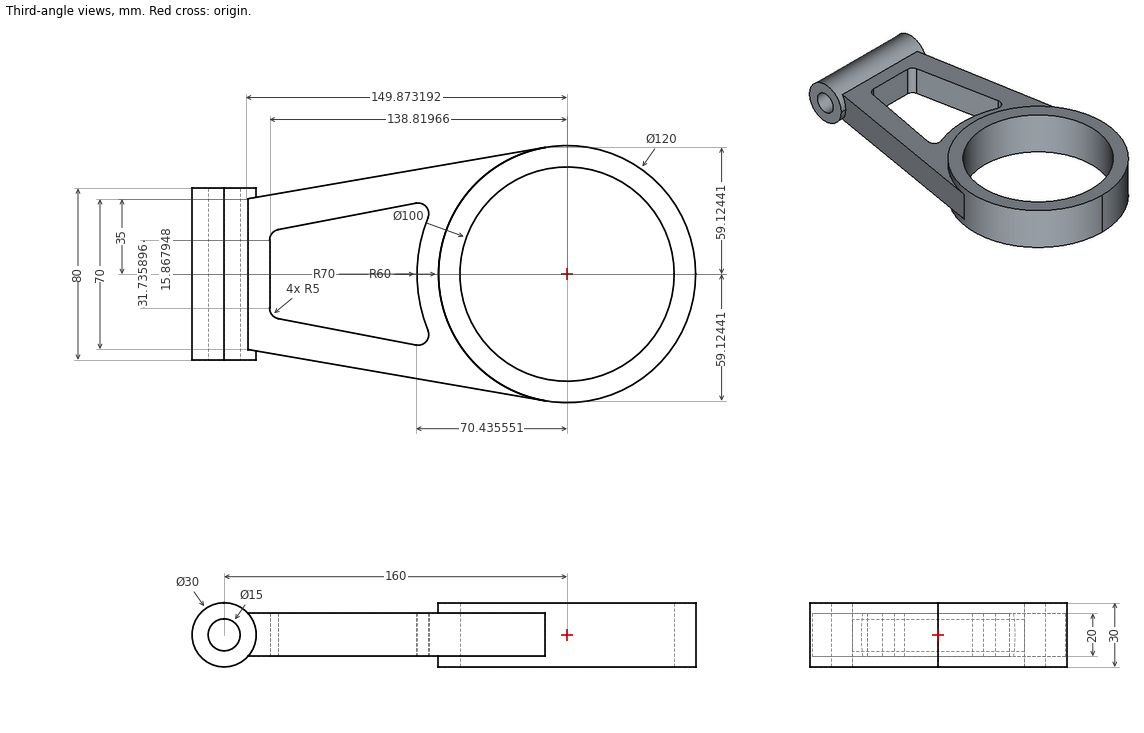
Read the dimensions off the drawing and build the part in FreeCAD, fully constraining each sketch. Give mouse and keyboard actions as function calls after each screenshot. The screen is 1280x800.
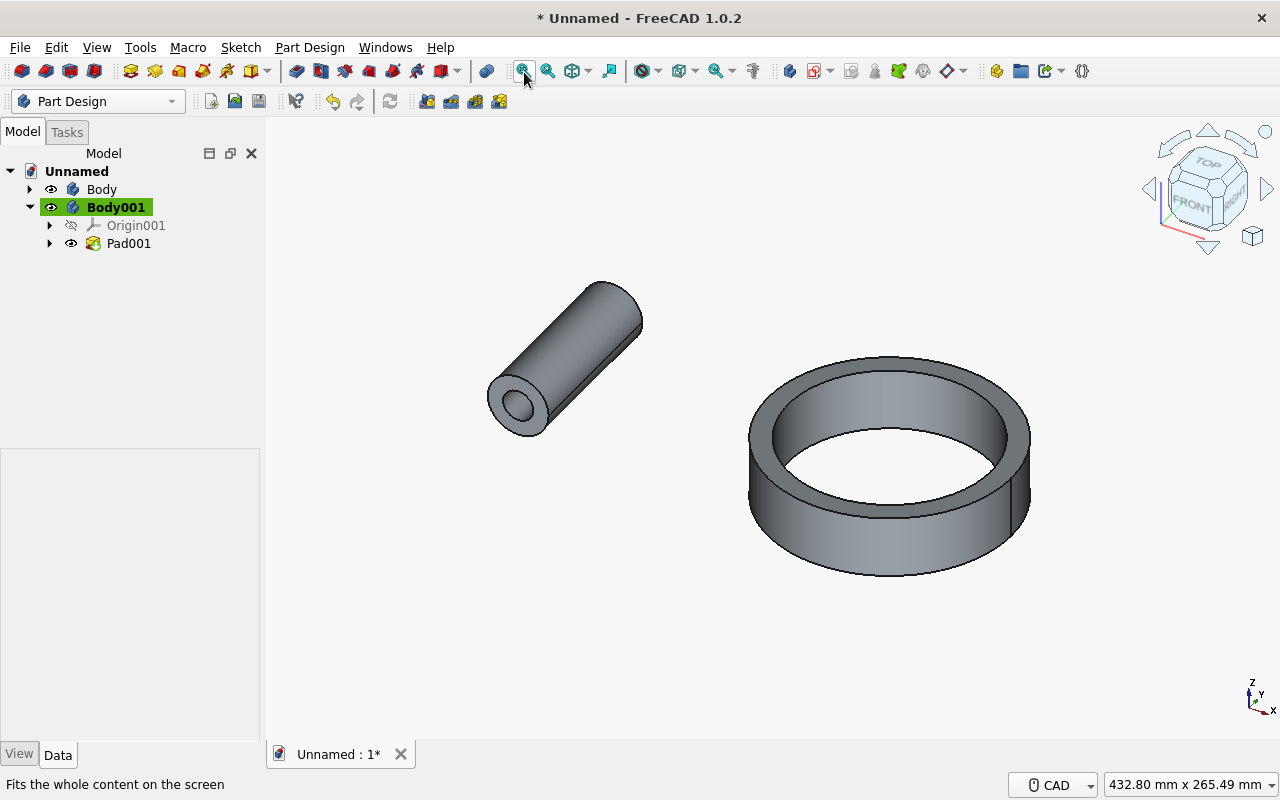
double_click(96, 189)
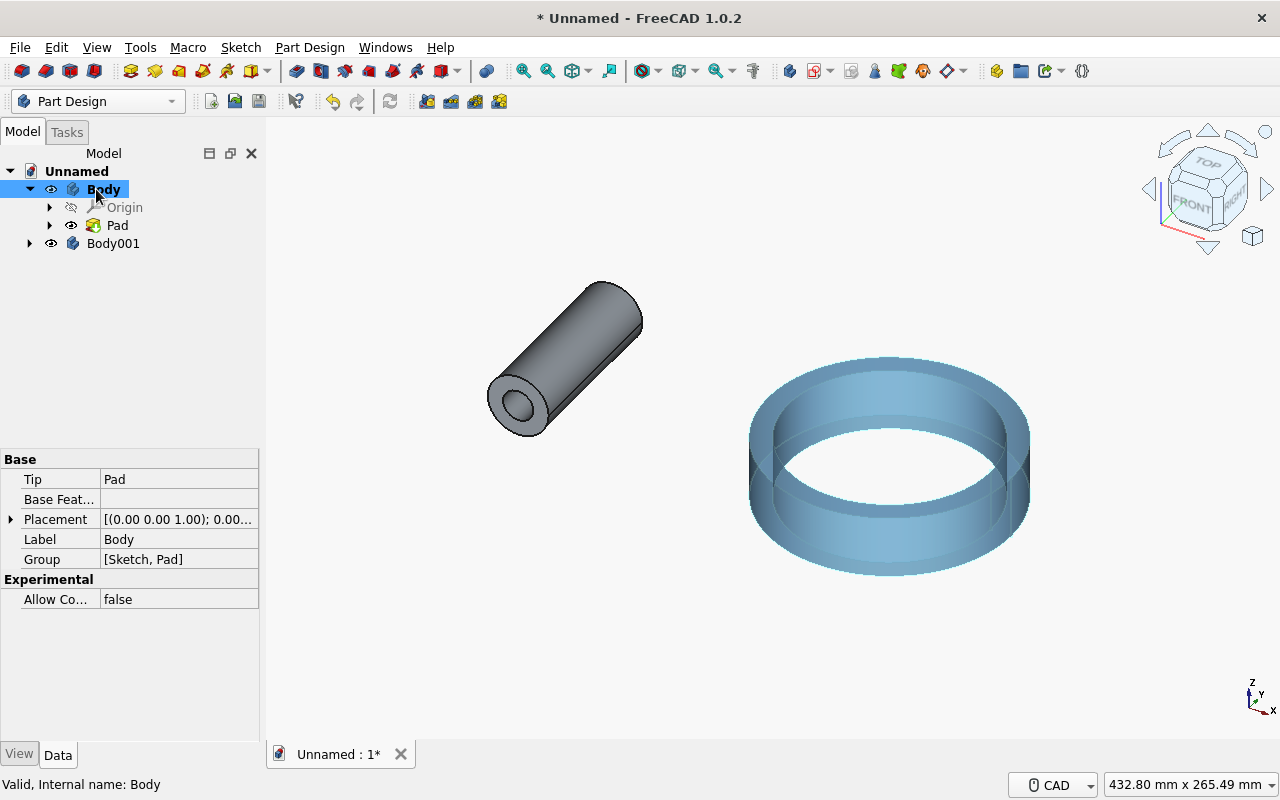
click(96, 189)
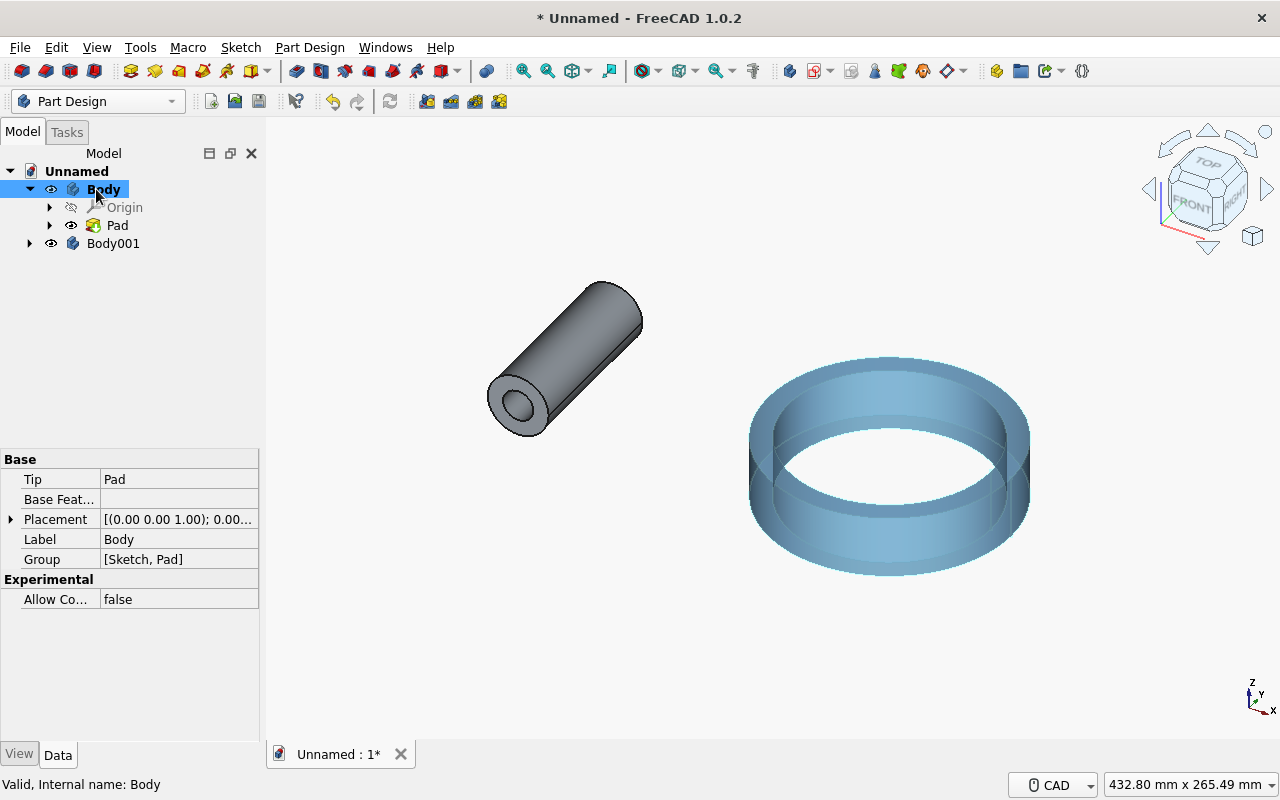
click(146, 599)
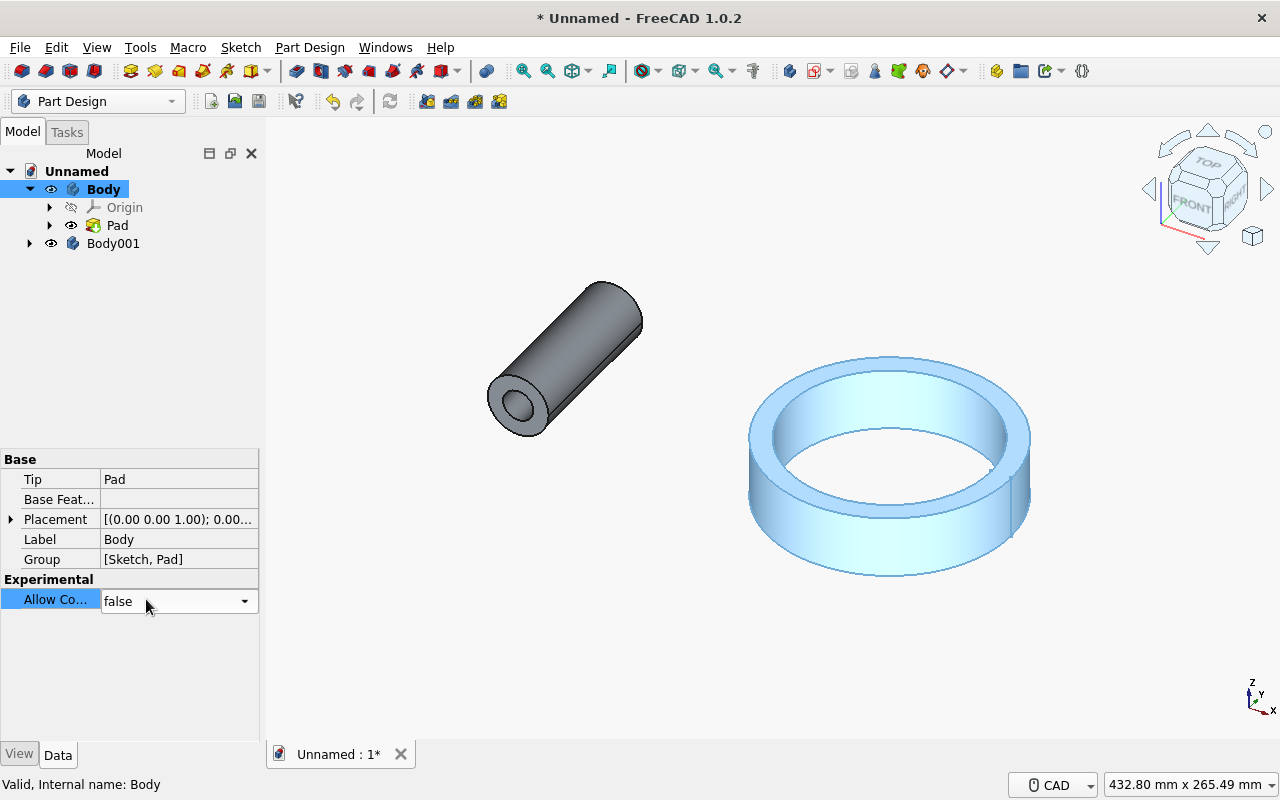
click(146, 599)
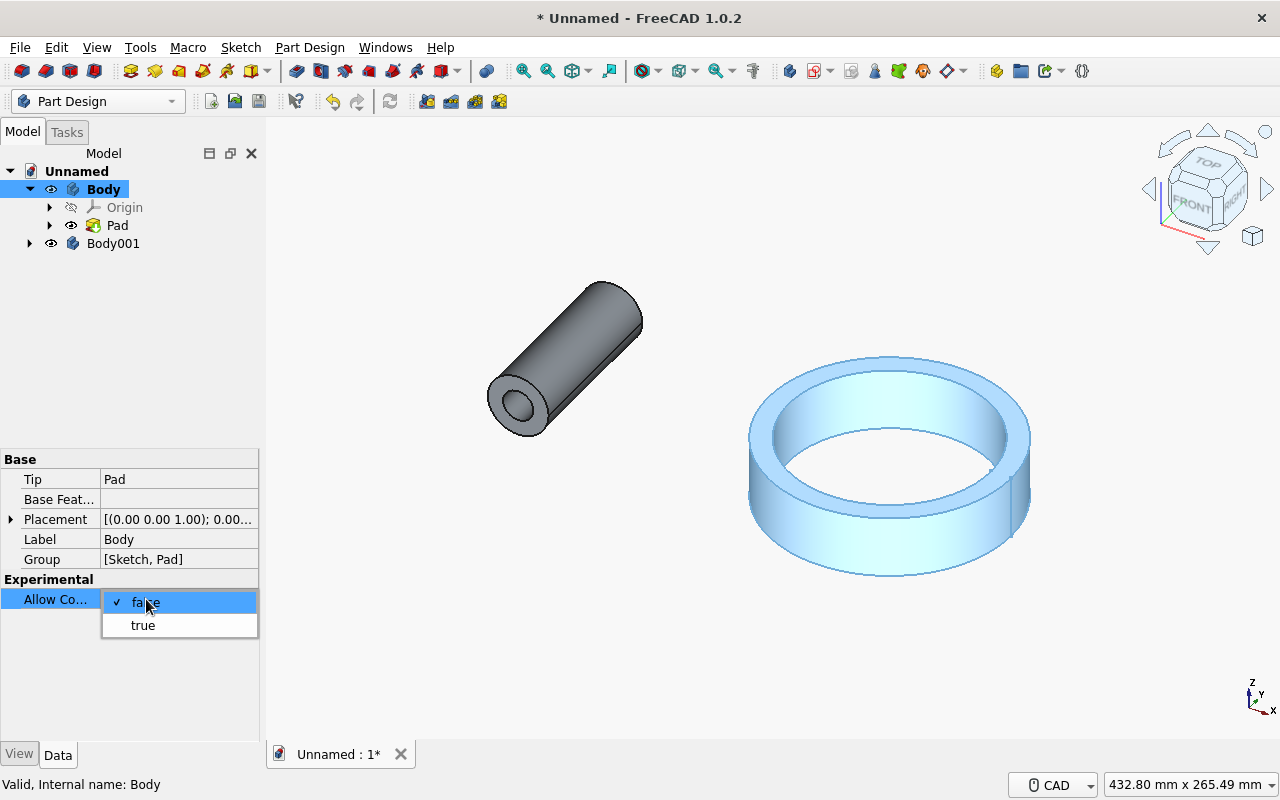
click(179, 626)
key(Return)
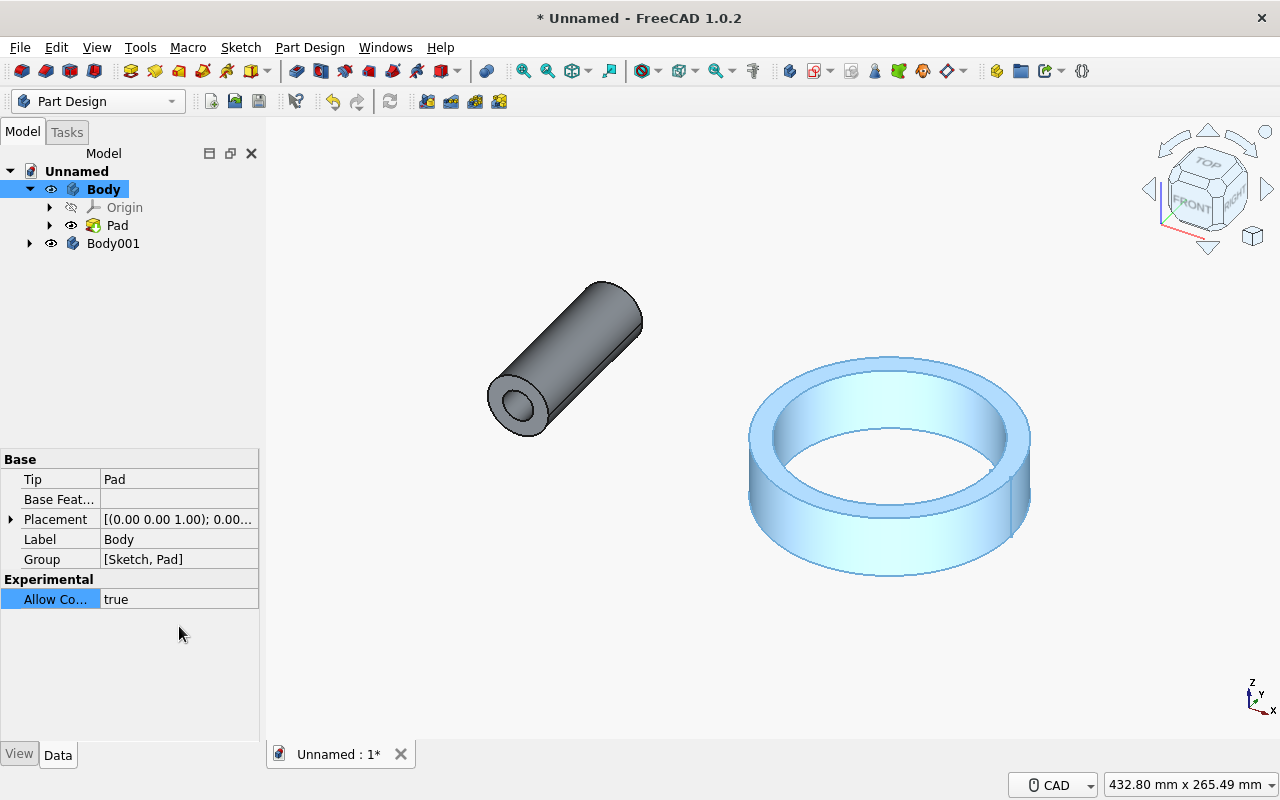
click(96, 243)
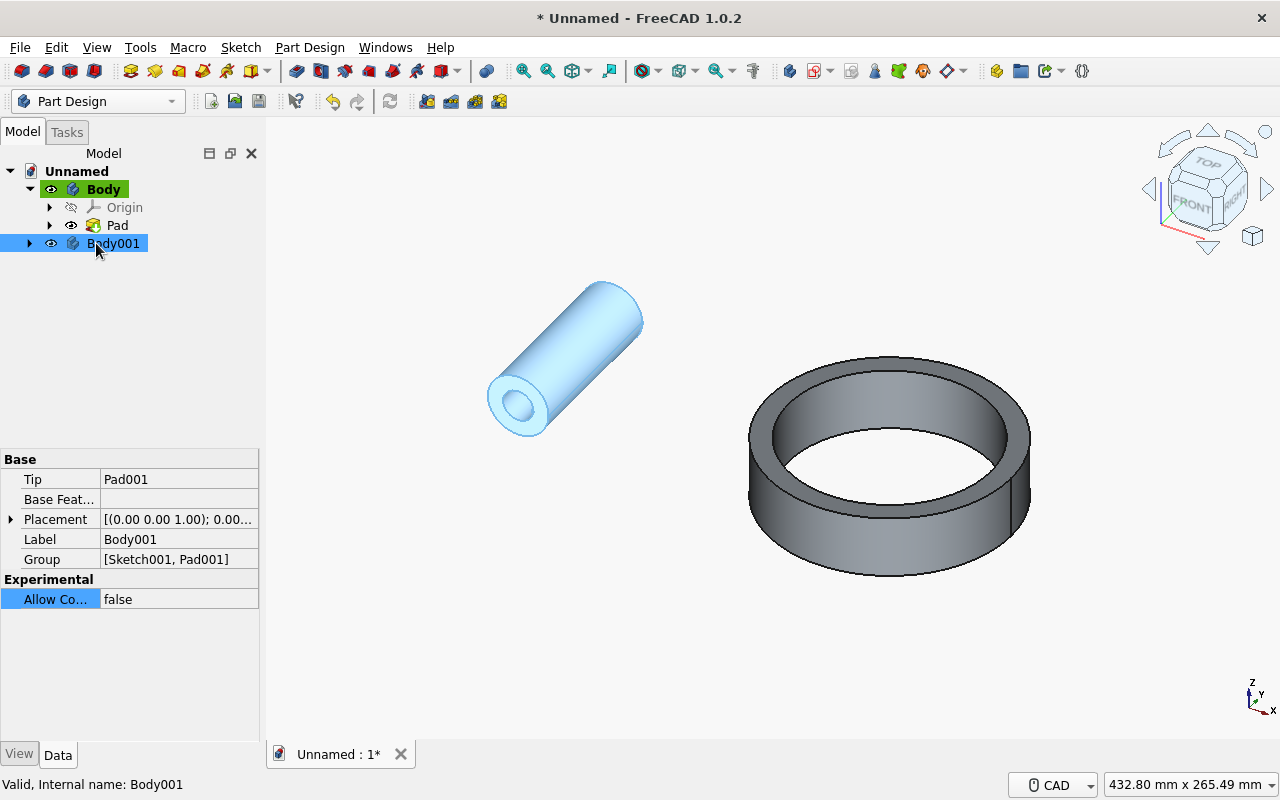
click(488, 72)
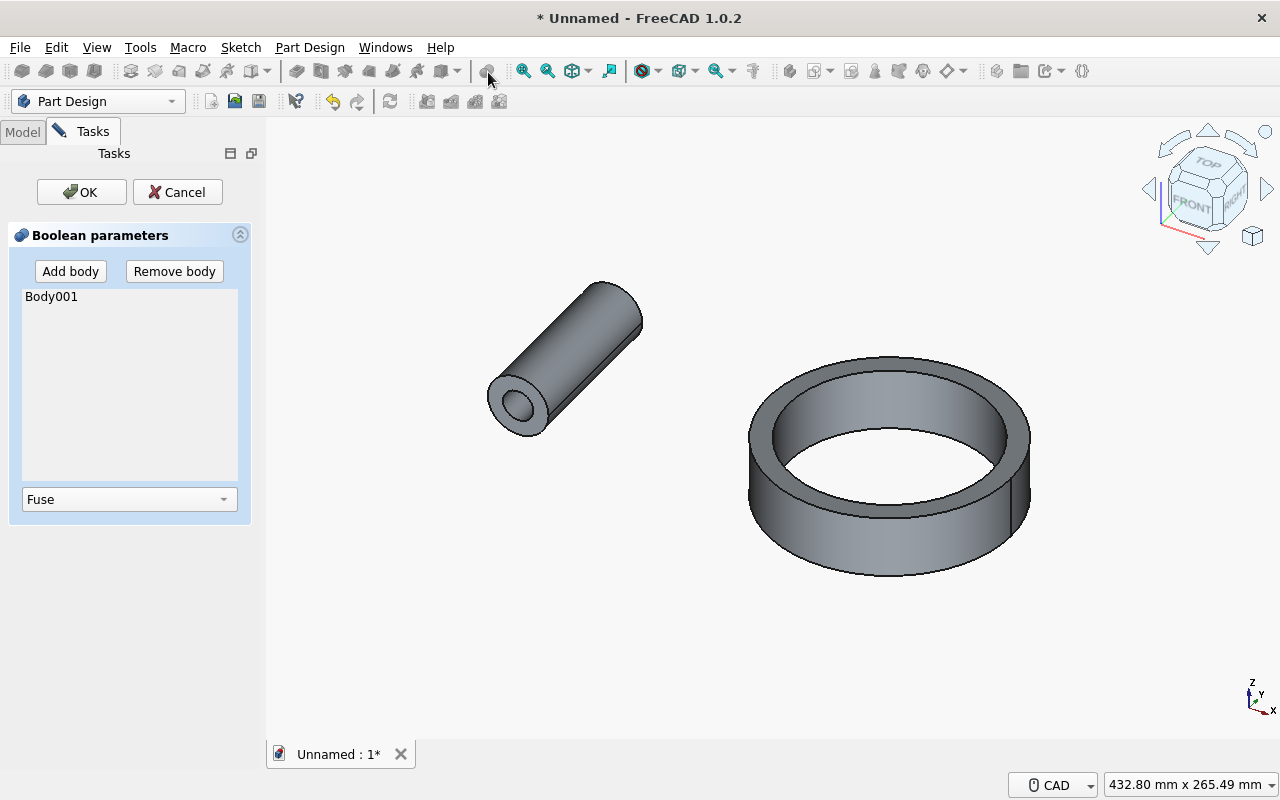
click(82, 192)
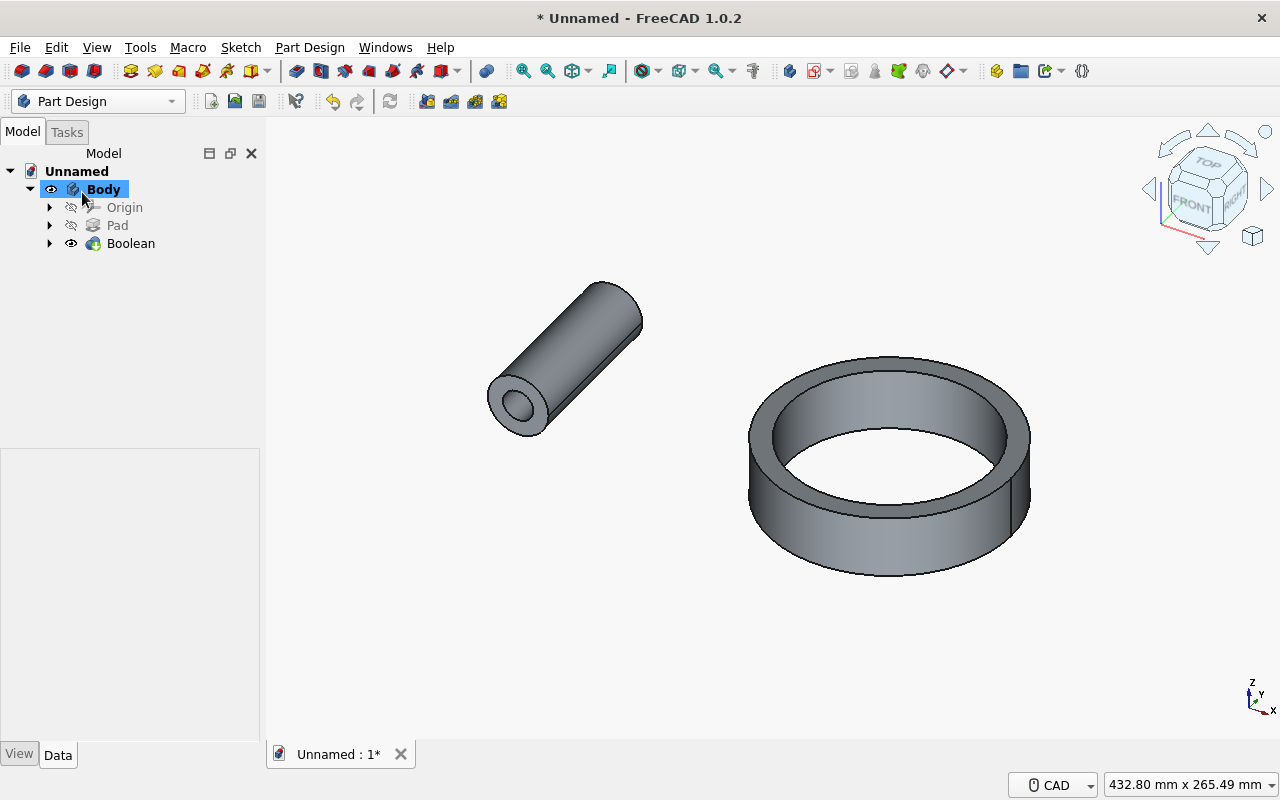
click(814, 72)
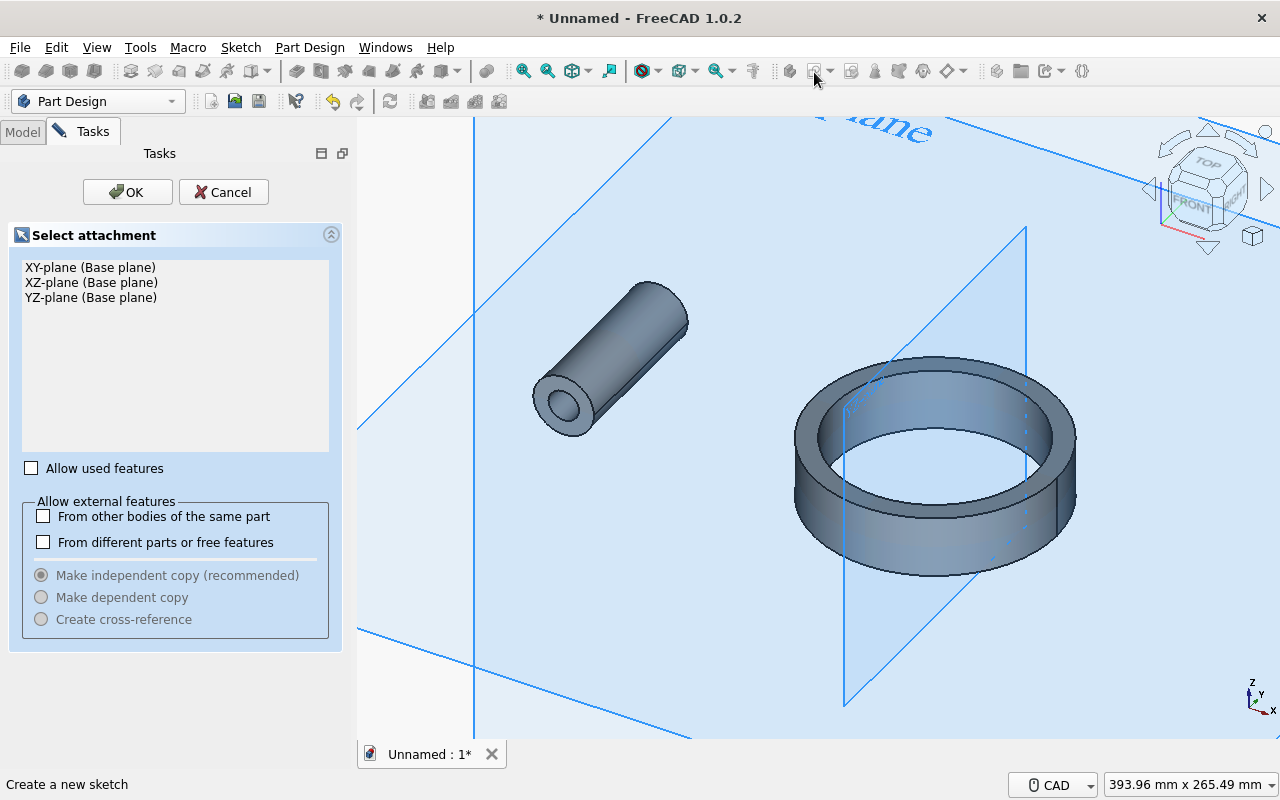
click(82, 268)